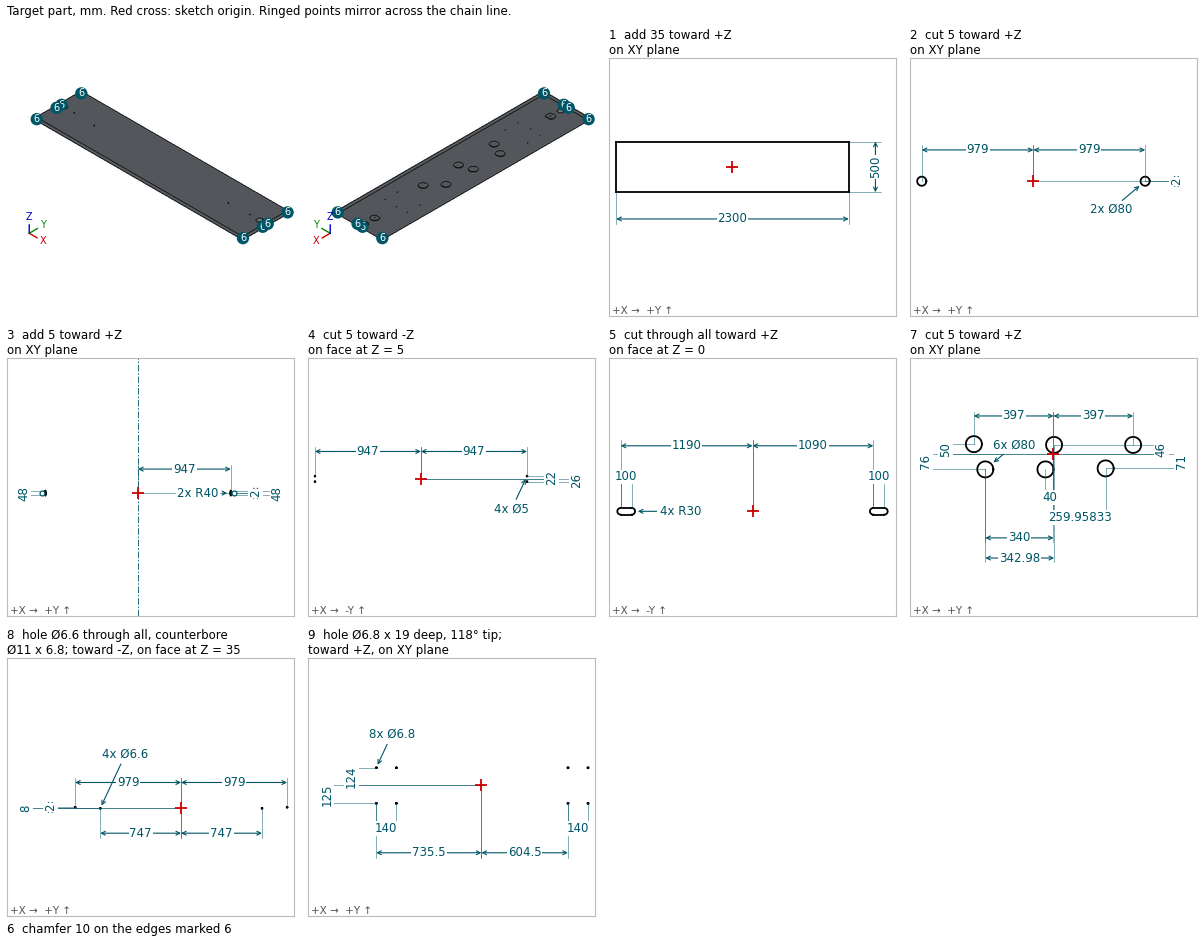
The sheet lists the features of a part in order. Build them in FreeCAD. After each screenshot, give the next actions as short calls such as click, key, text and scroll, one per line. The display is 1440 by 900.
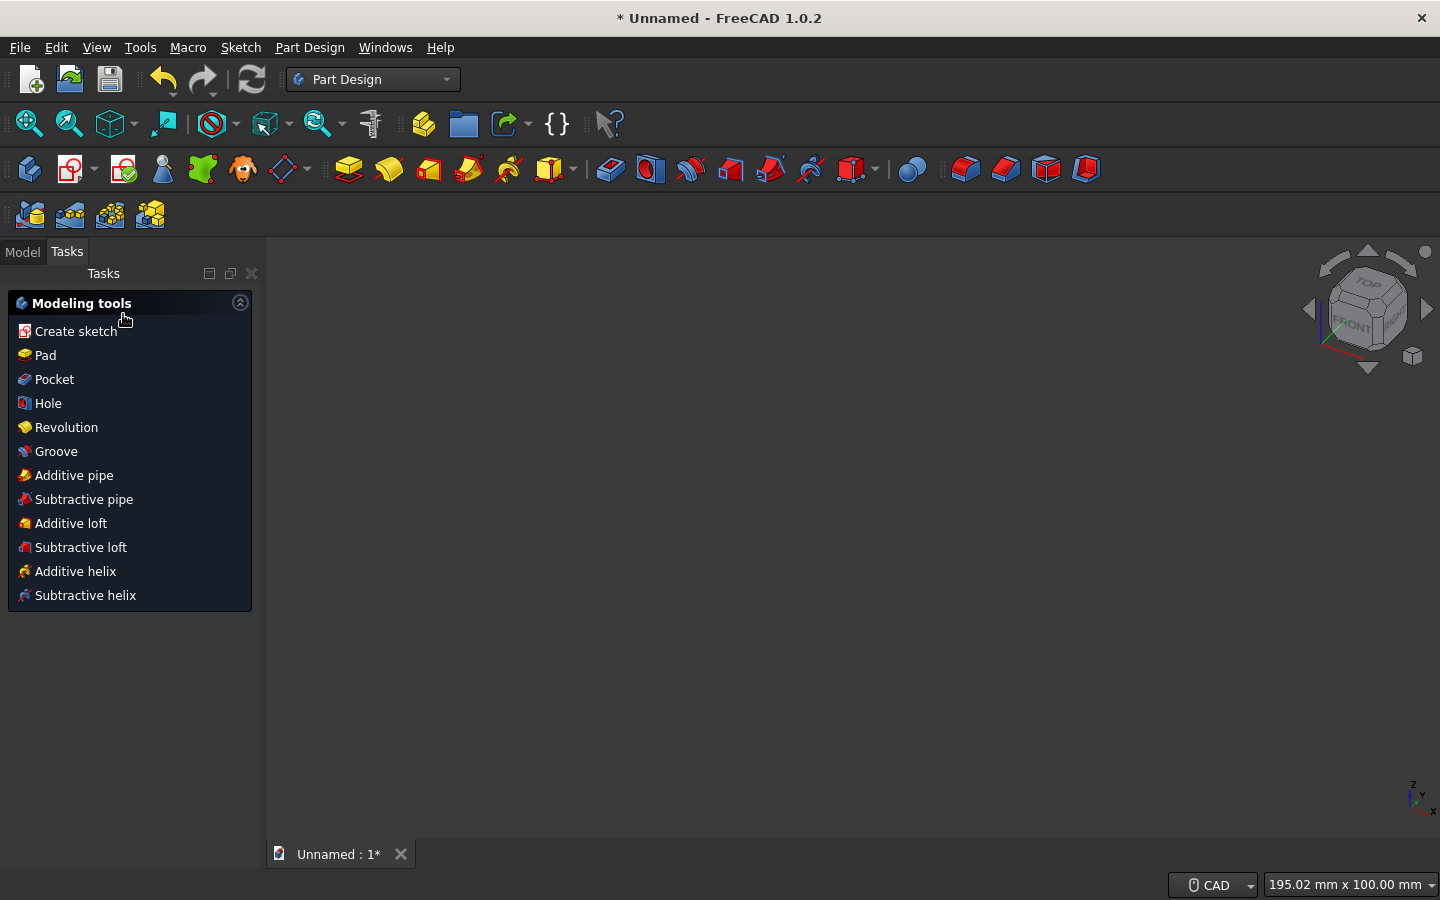
click(350, 170)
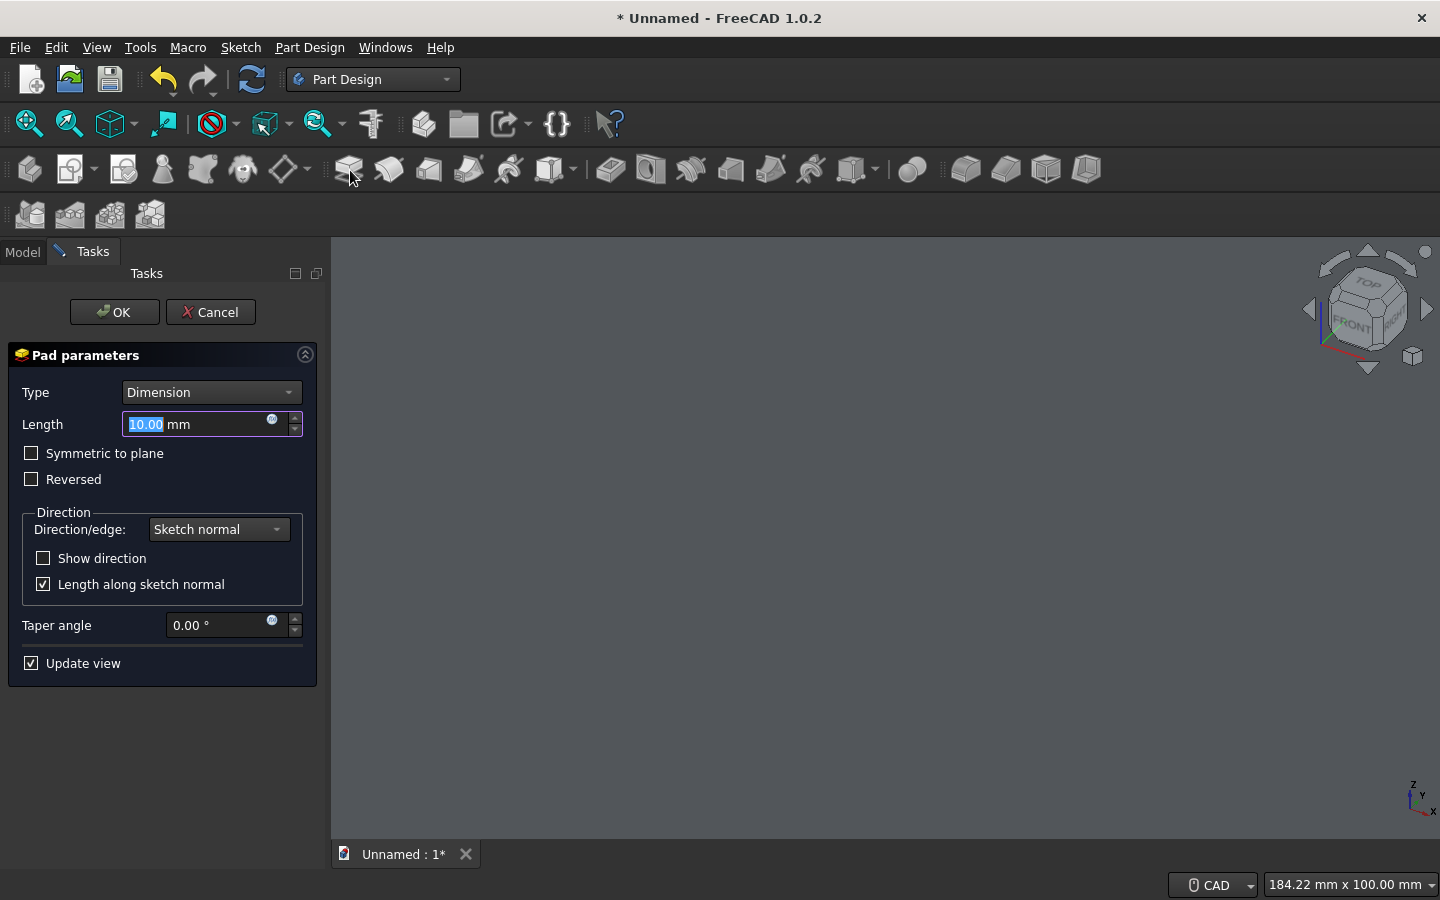
text(35)
key(Tab)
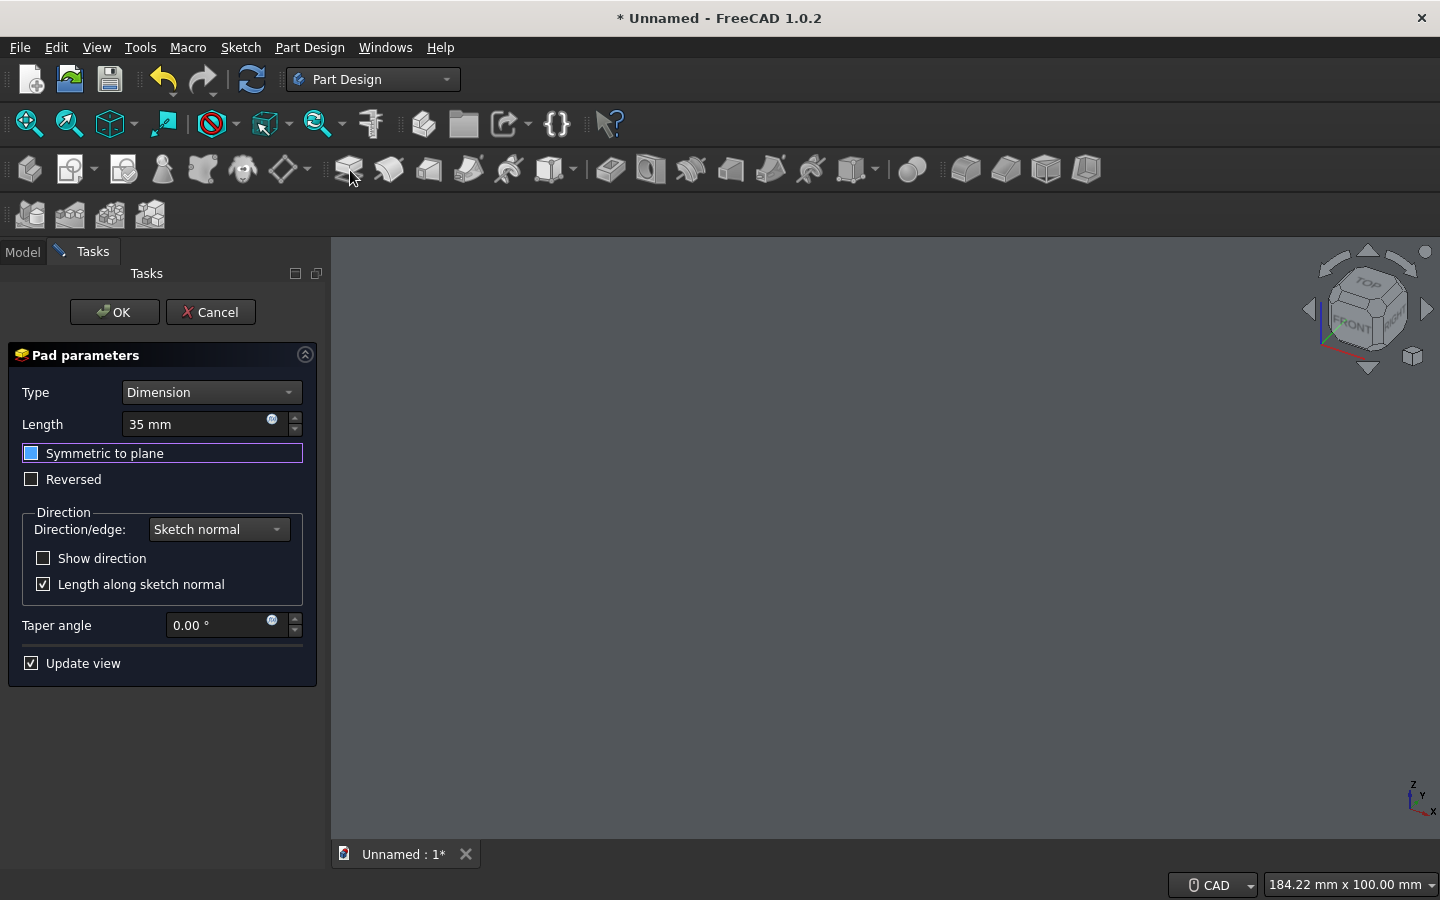
click(115, 312)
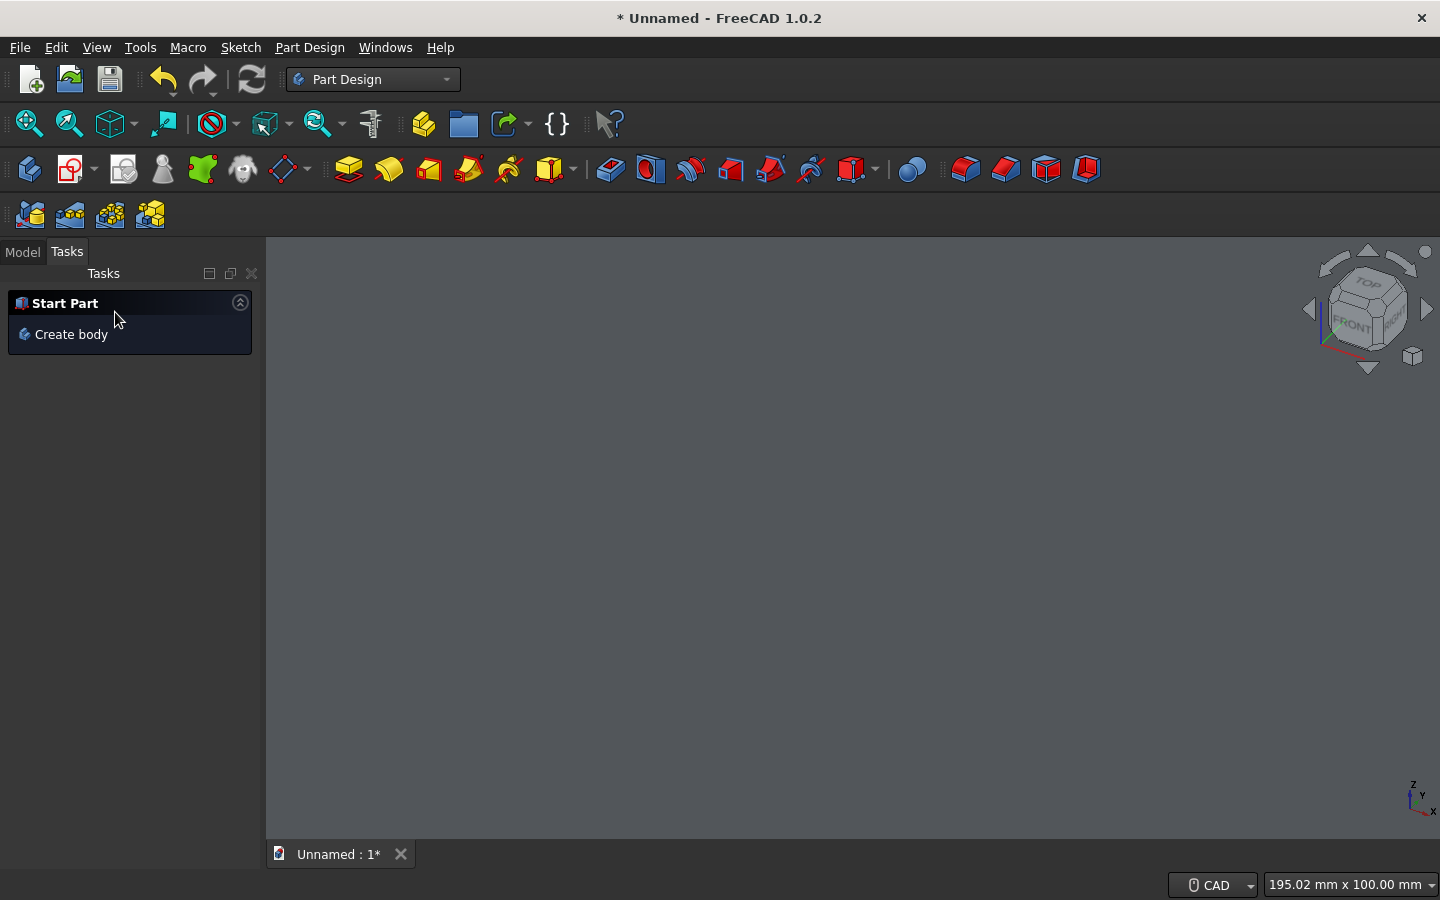
click(30, 124)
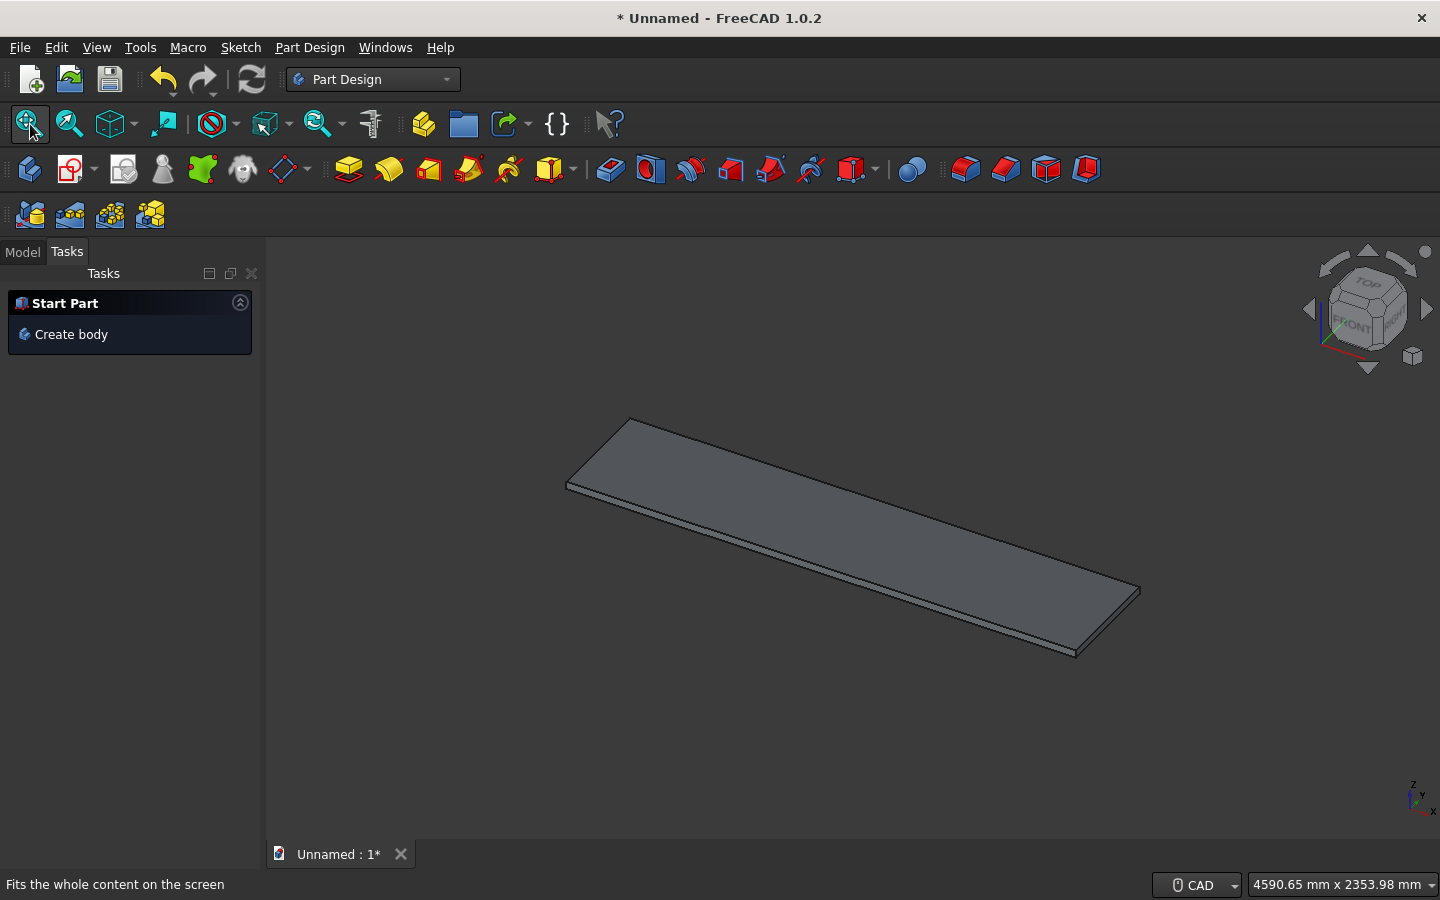
click(70, 170)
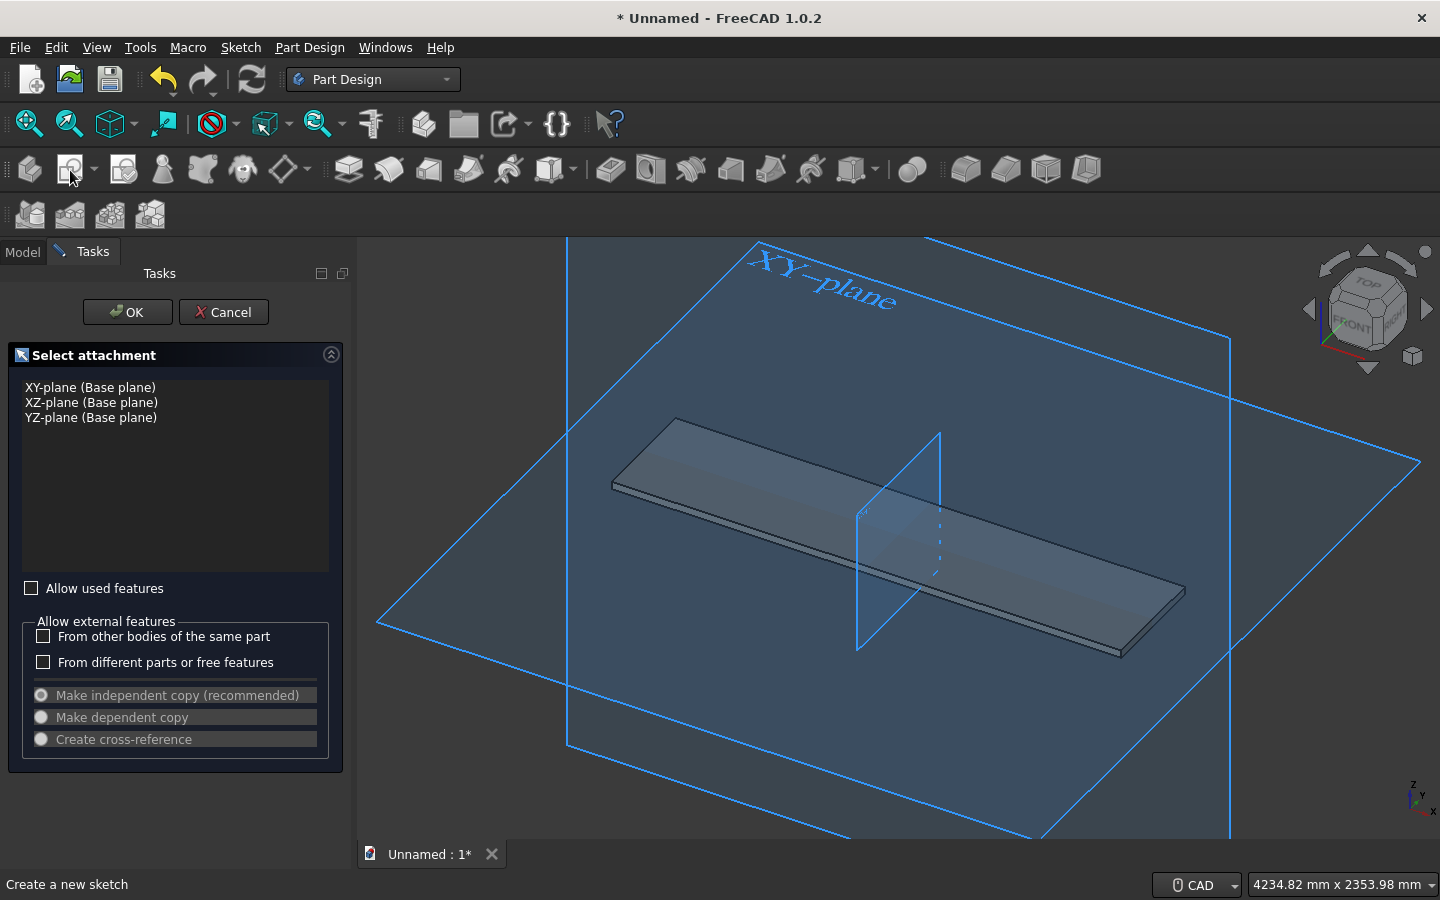
click(82, 388)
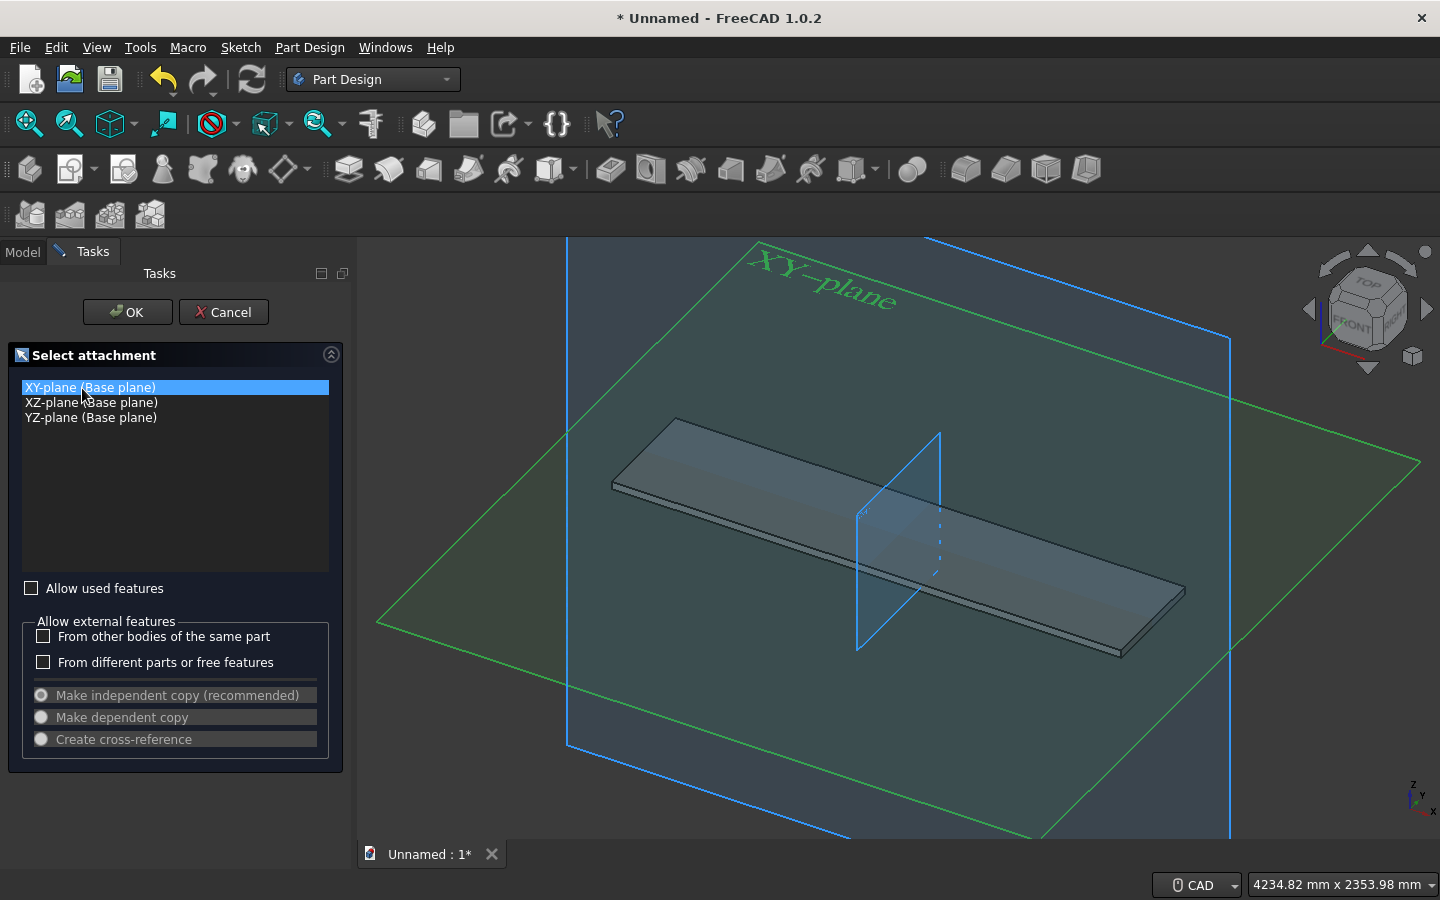
click(128, 312)